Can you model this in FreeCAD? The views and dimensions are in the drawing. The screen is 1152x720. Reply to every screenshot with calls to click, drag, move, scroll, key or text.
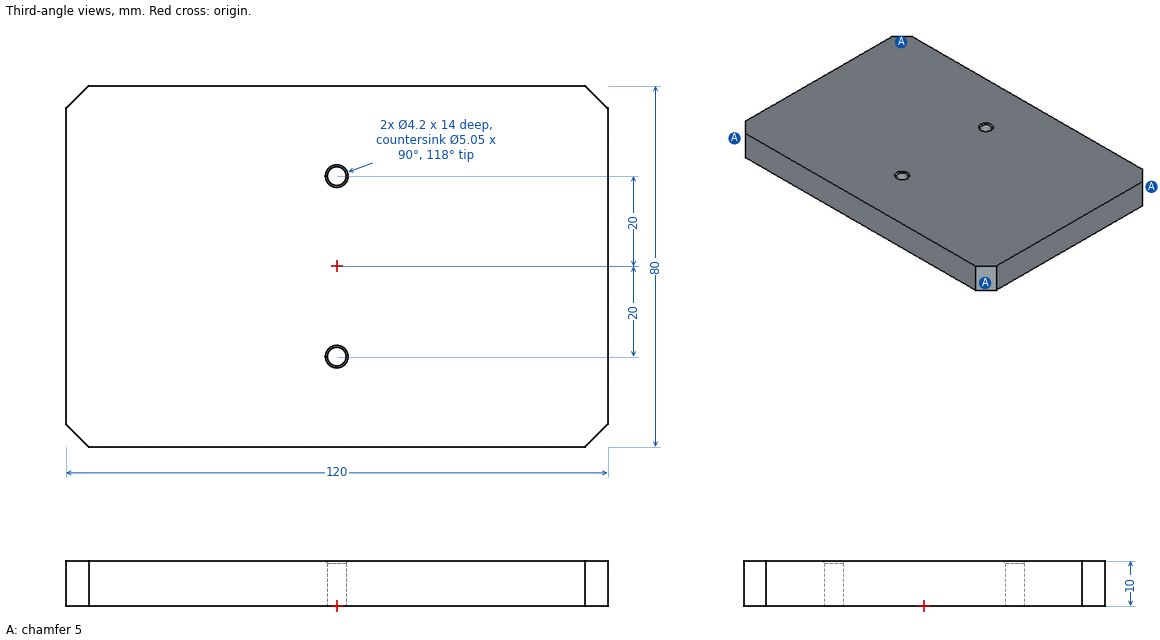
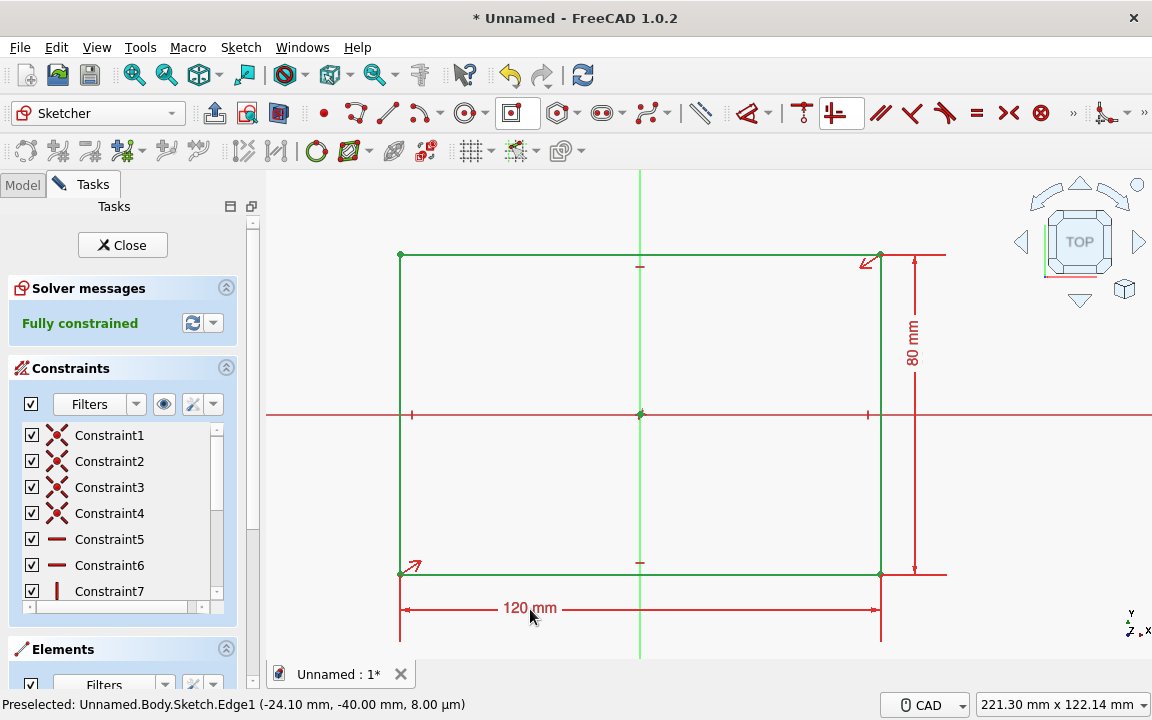
click(123, 245)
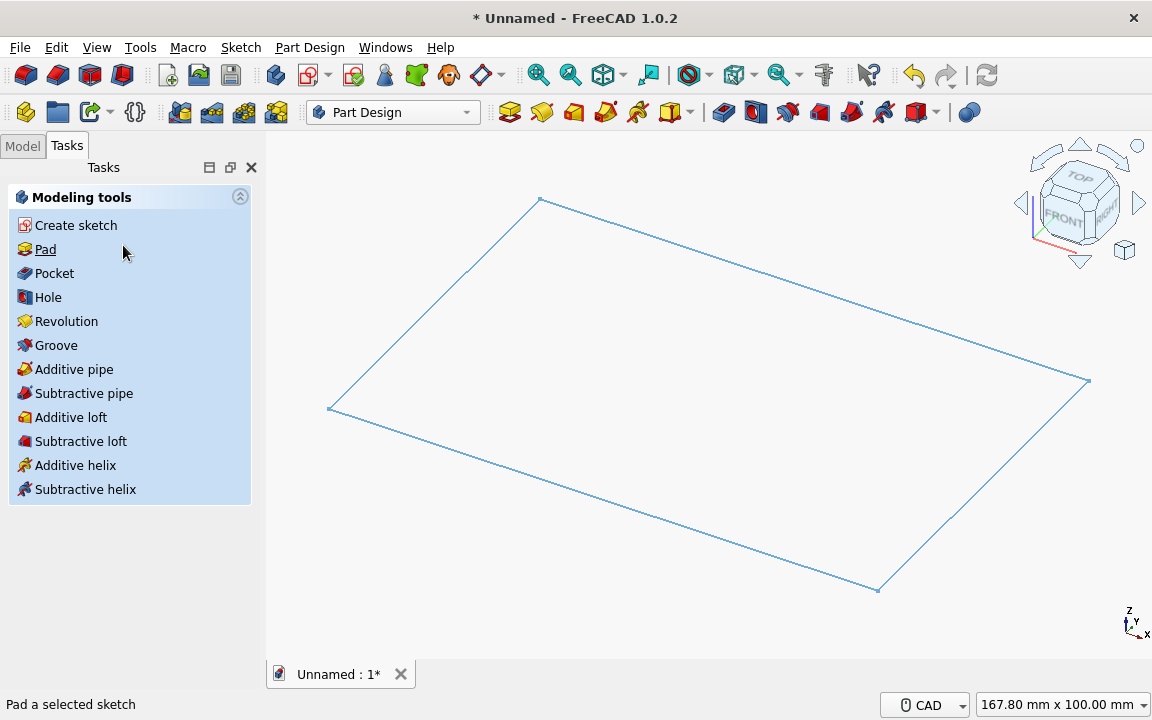
click(510, 112)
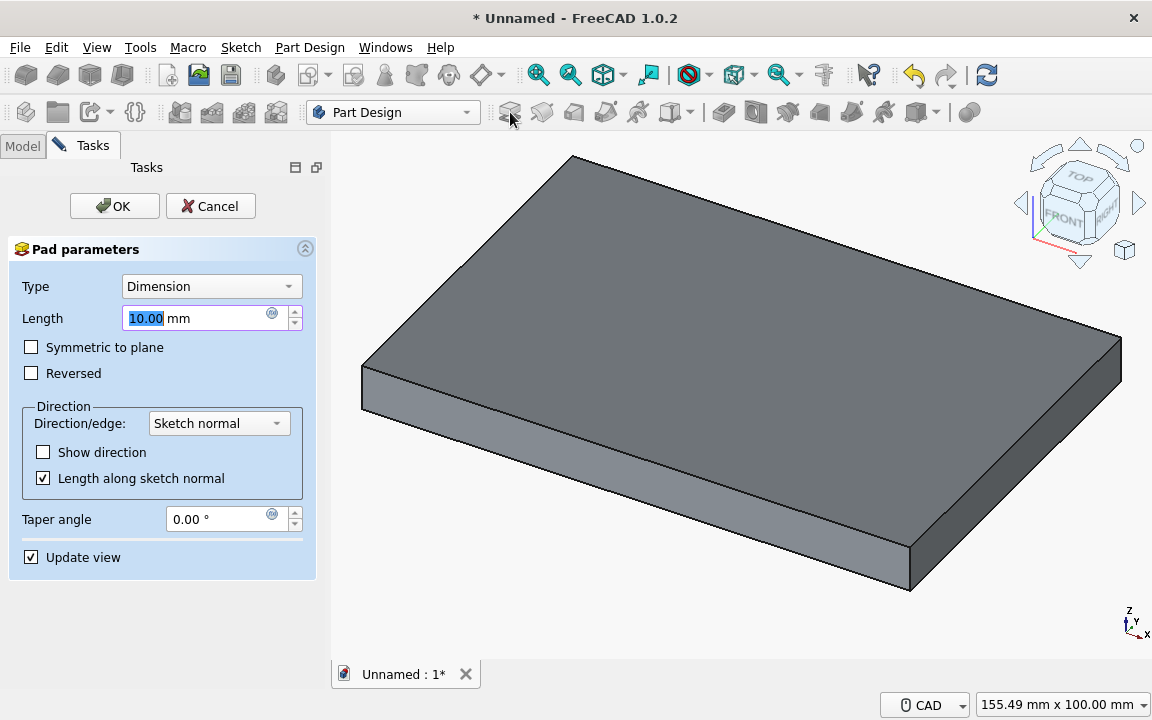
text(10)
key(Tab)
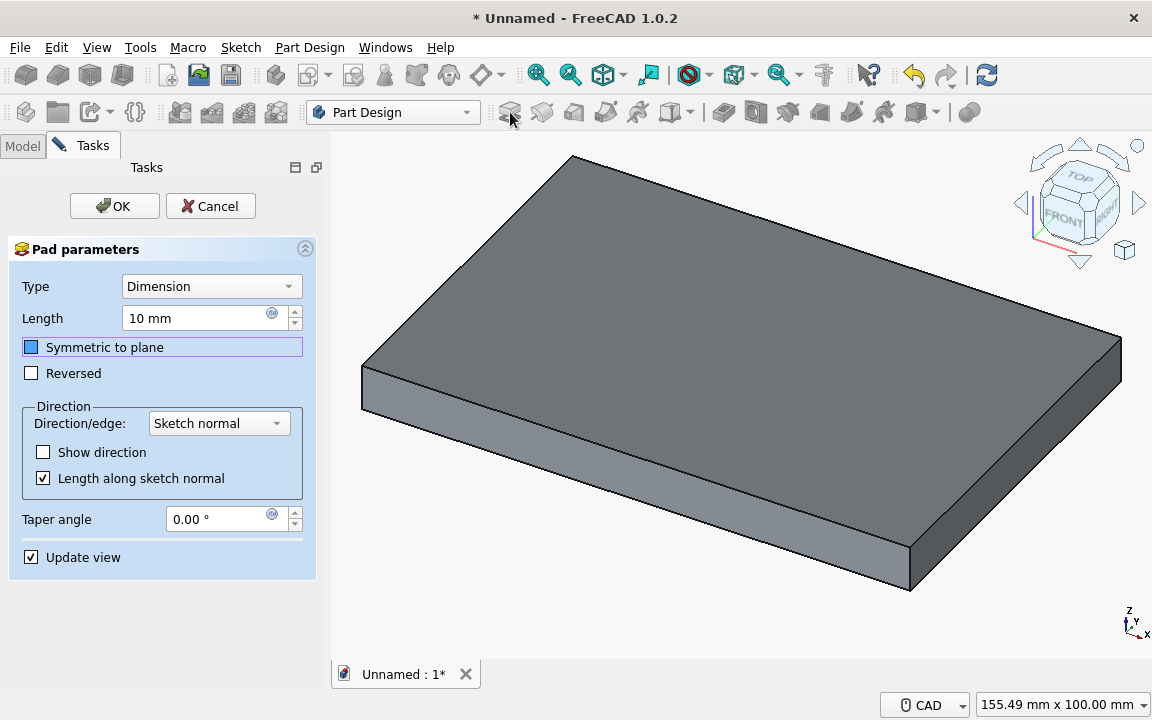
click(115, 206)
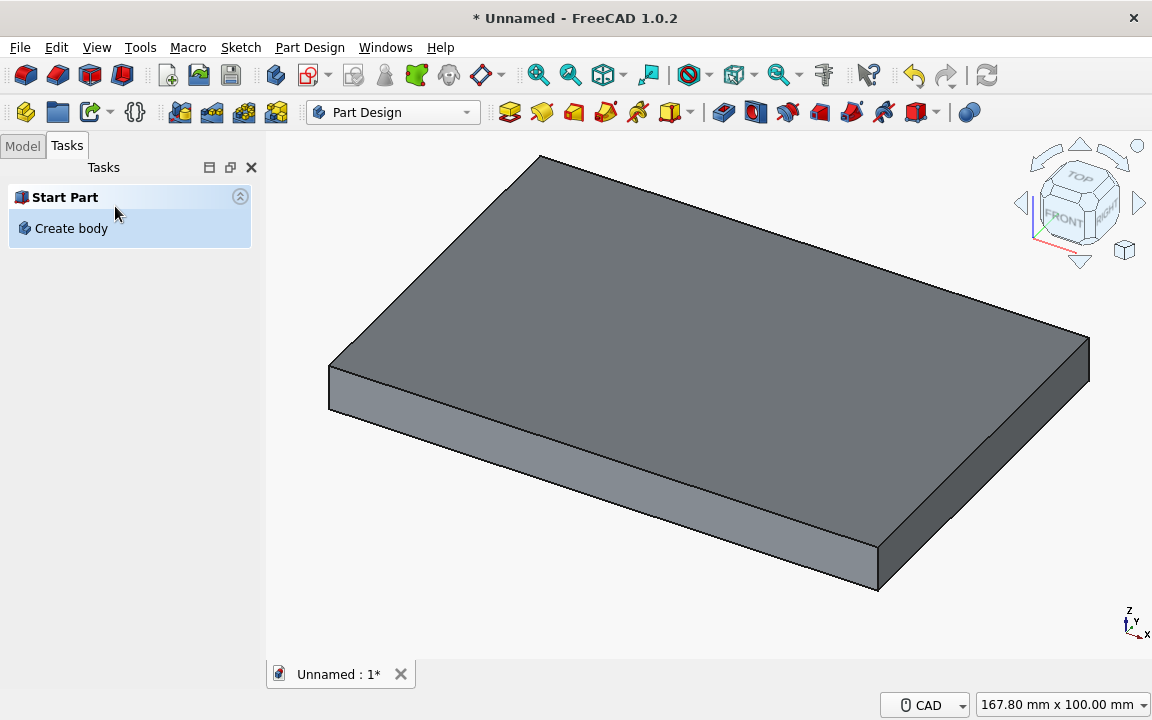
click(878, 568)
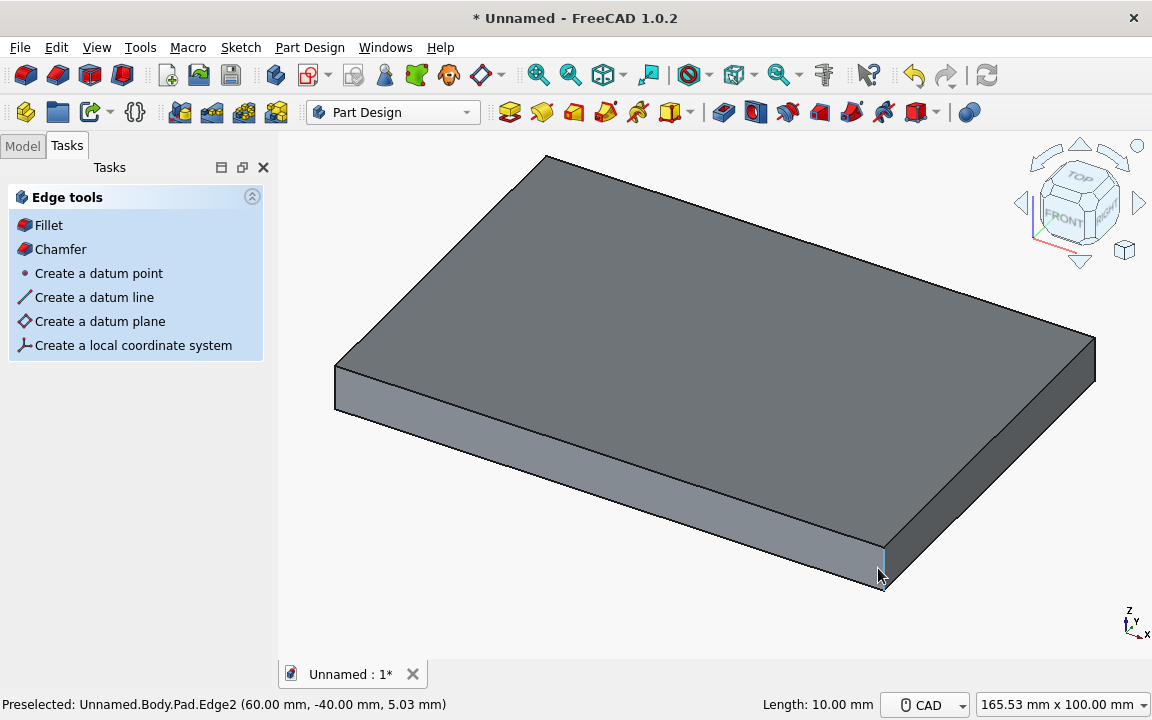
key(0)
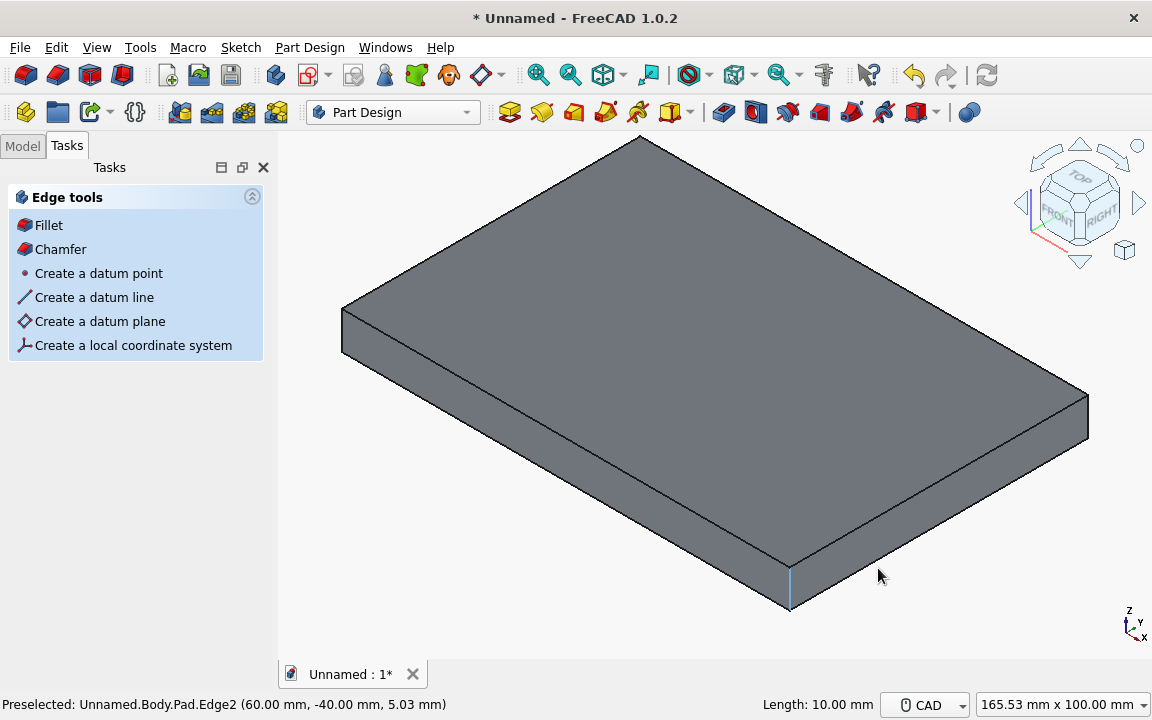
key(2)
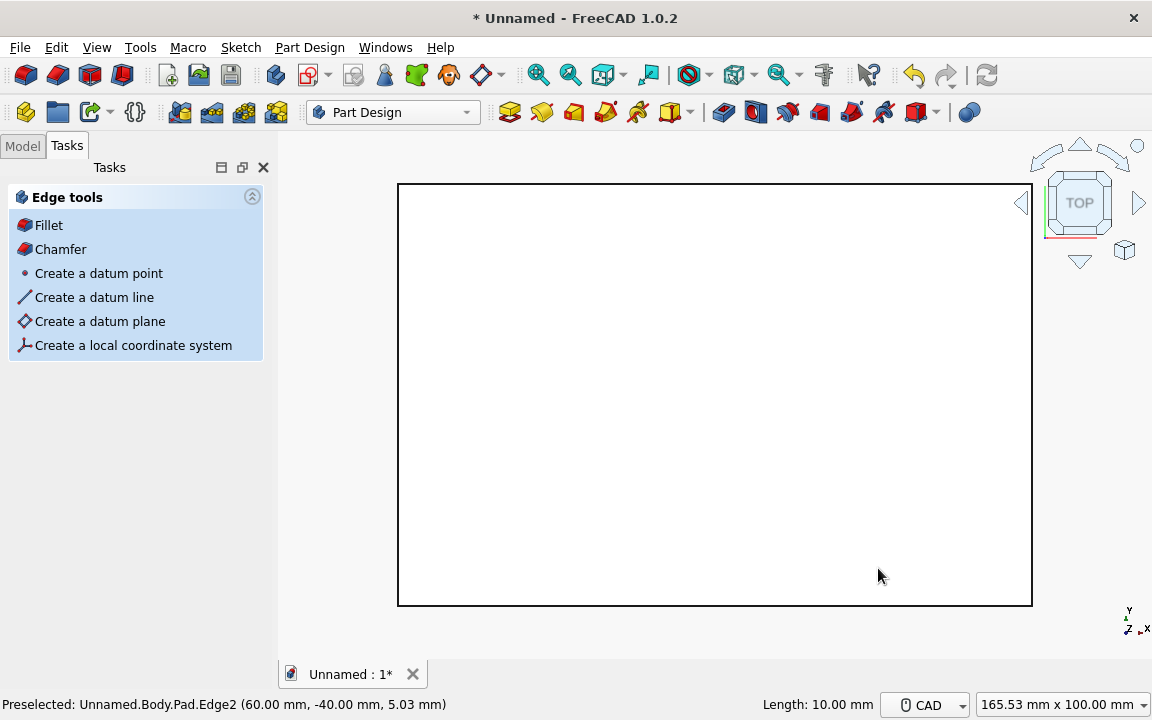
key(1)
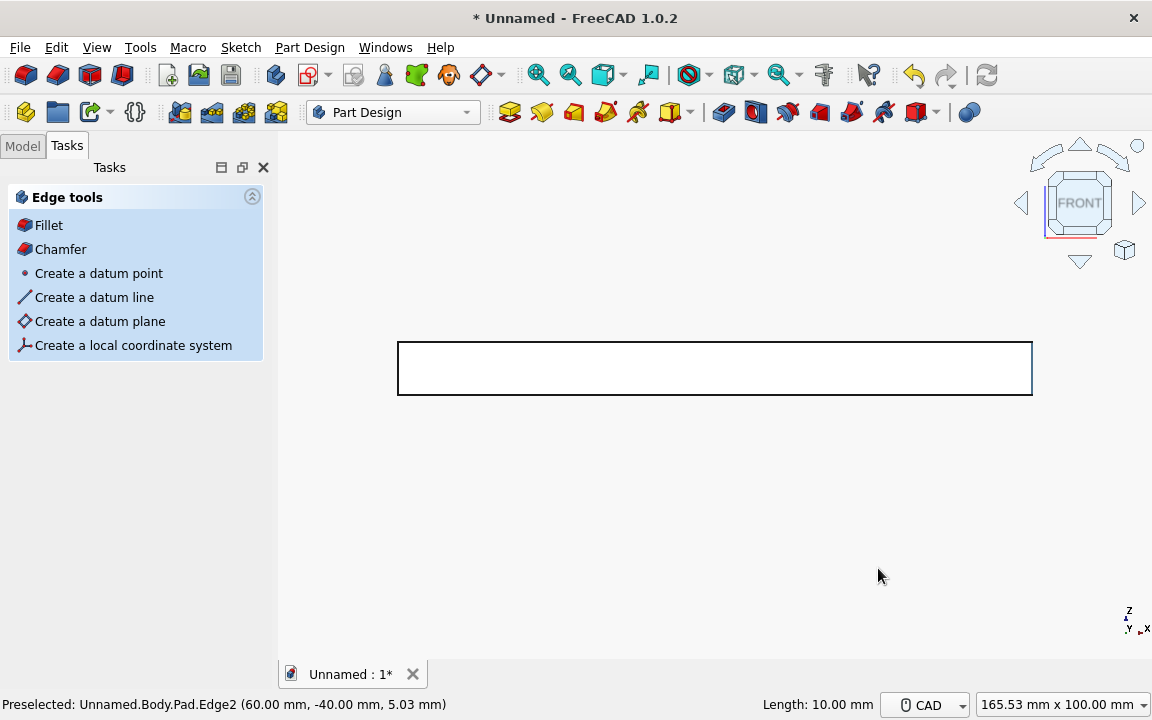
click(398, 368, ctrl)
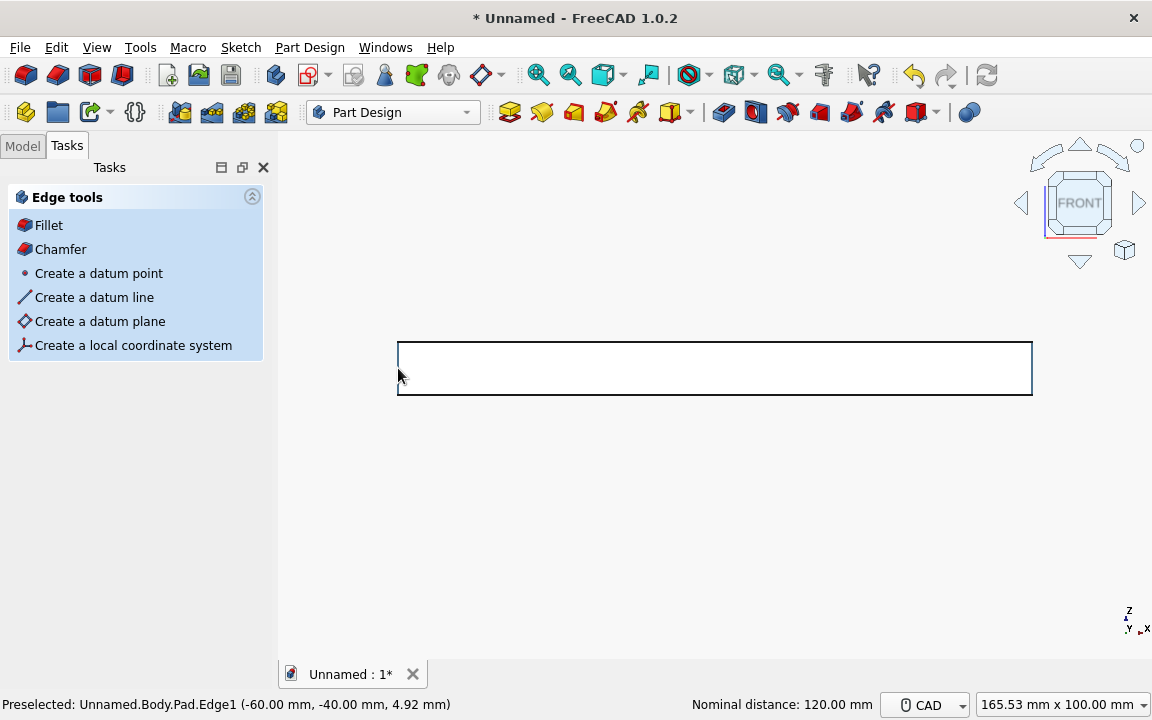
key(3)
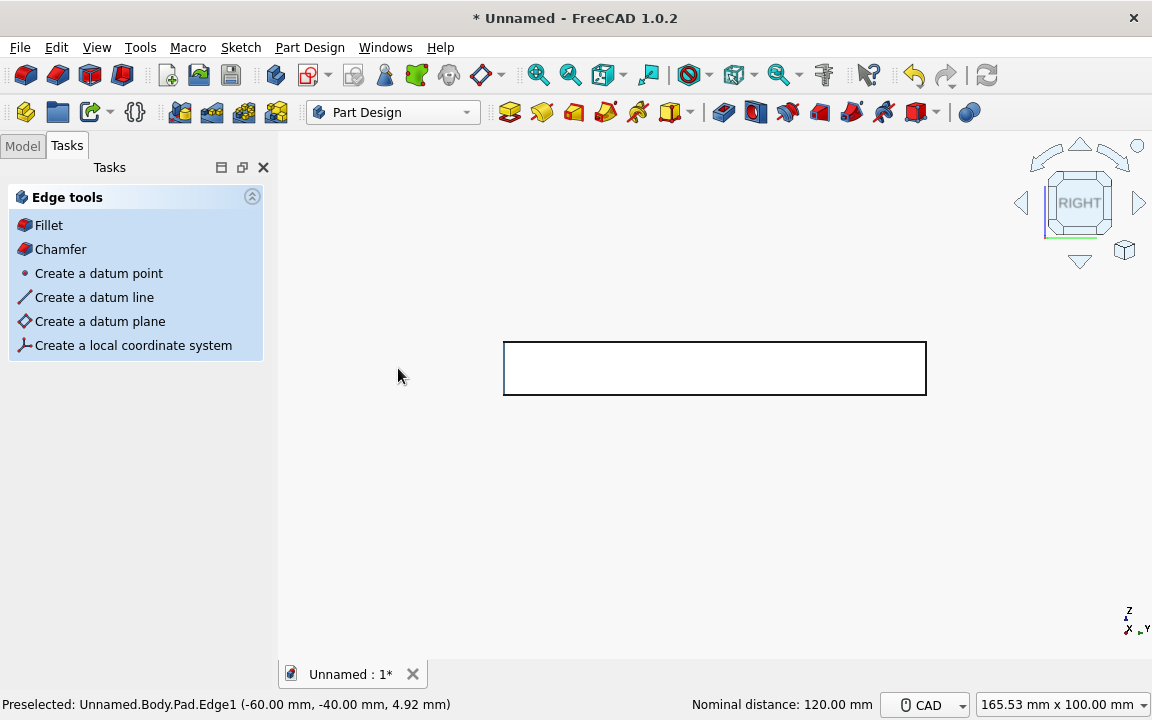
click(926, 368, ctrl)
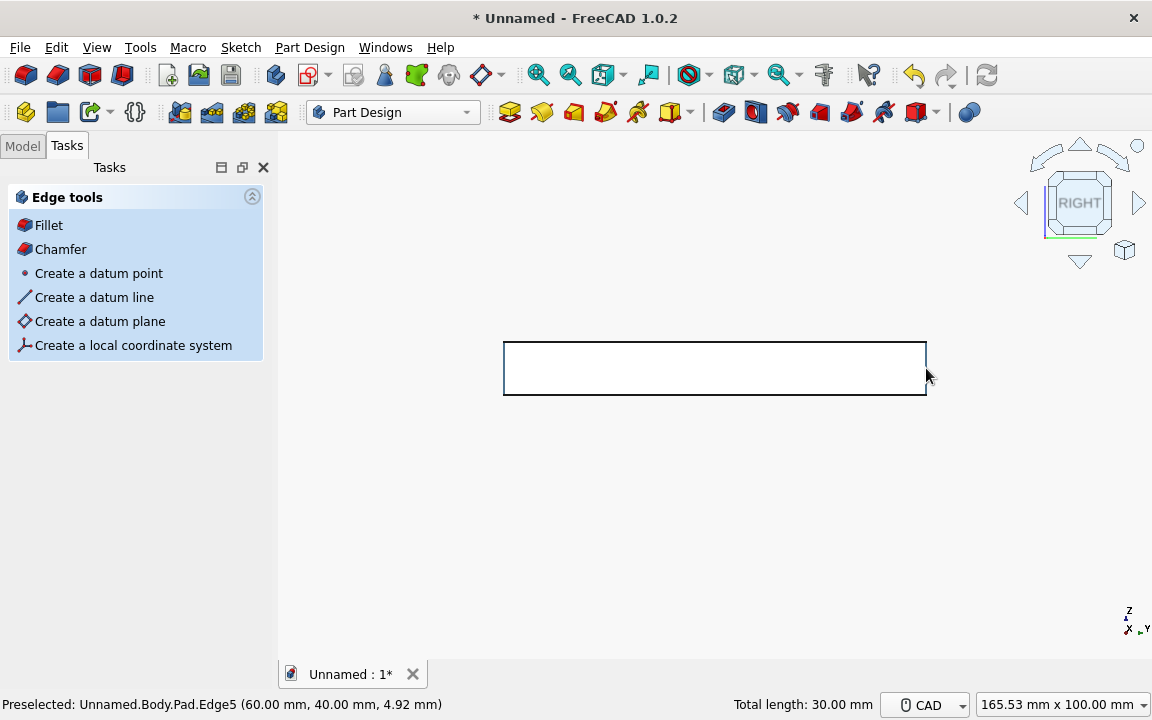
key(5)